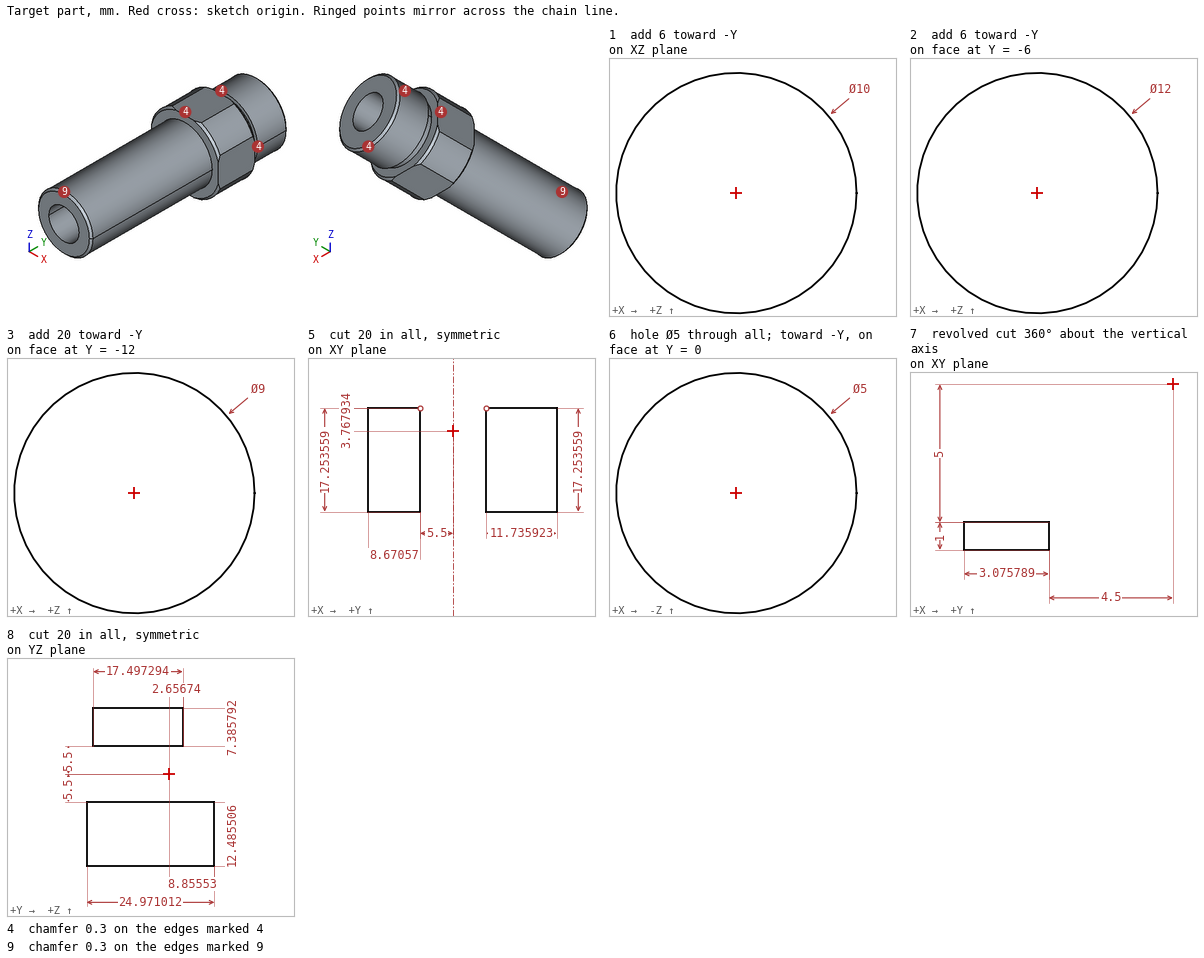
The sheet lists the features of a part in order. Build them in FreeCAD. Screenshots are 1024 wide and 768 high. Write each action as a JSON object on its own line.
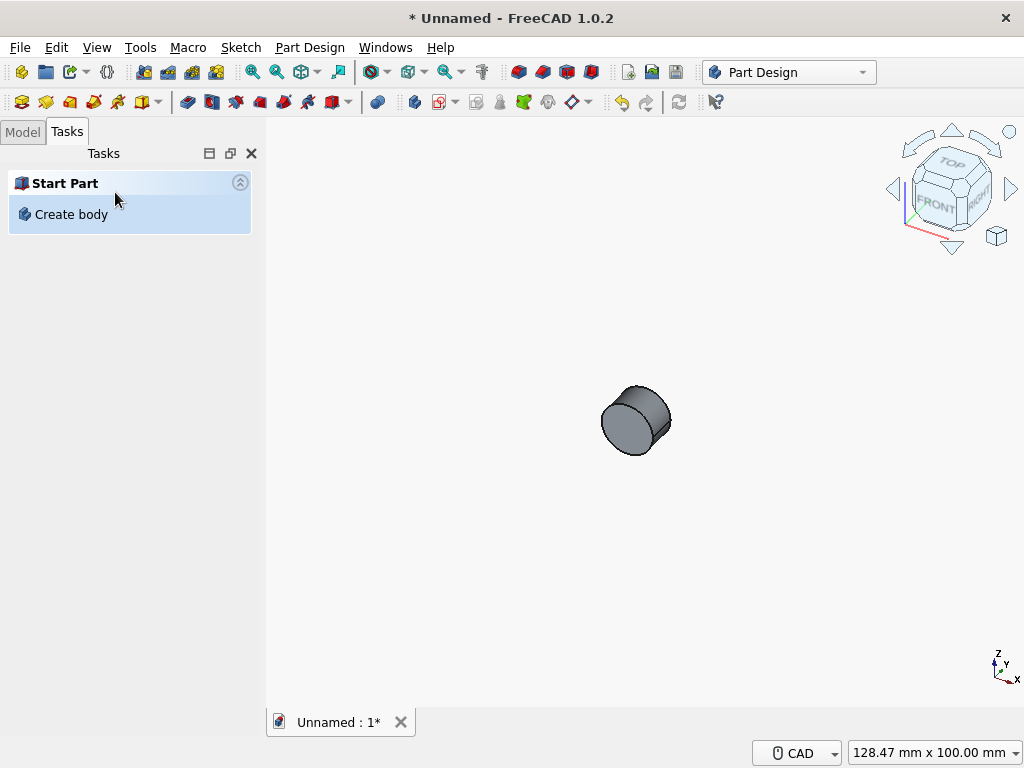
{"action": "key", "text": "v f"}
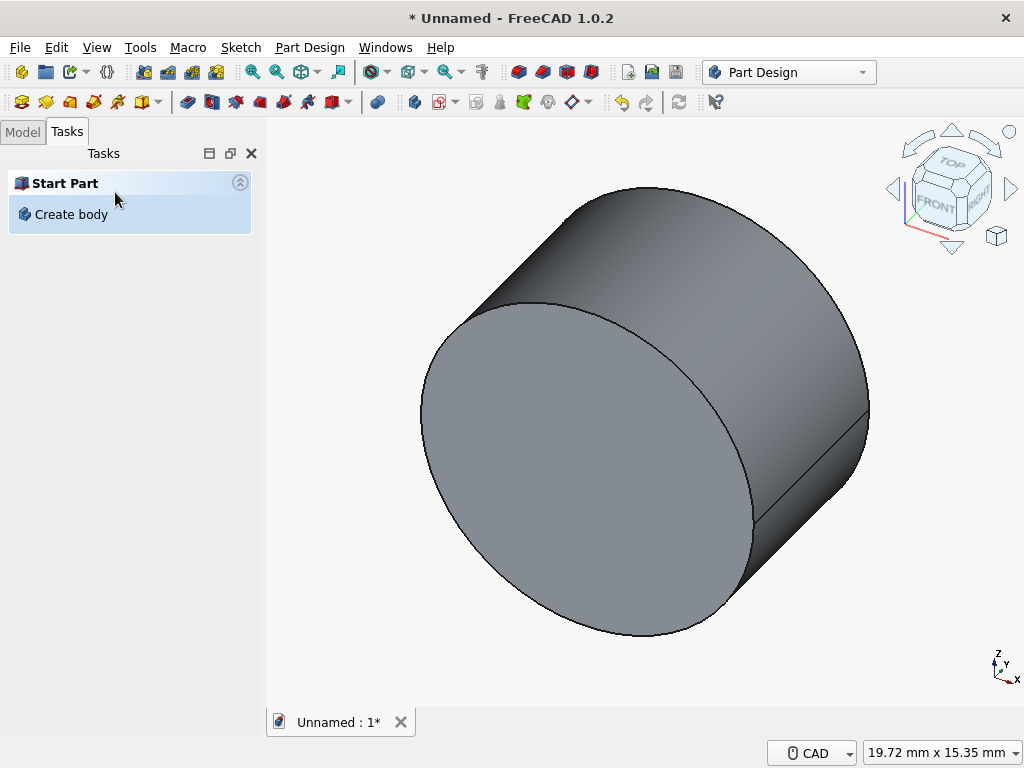
{"action": "left_click", "coordinate": [587, 468]}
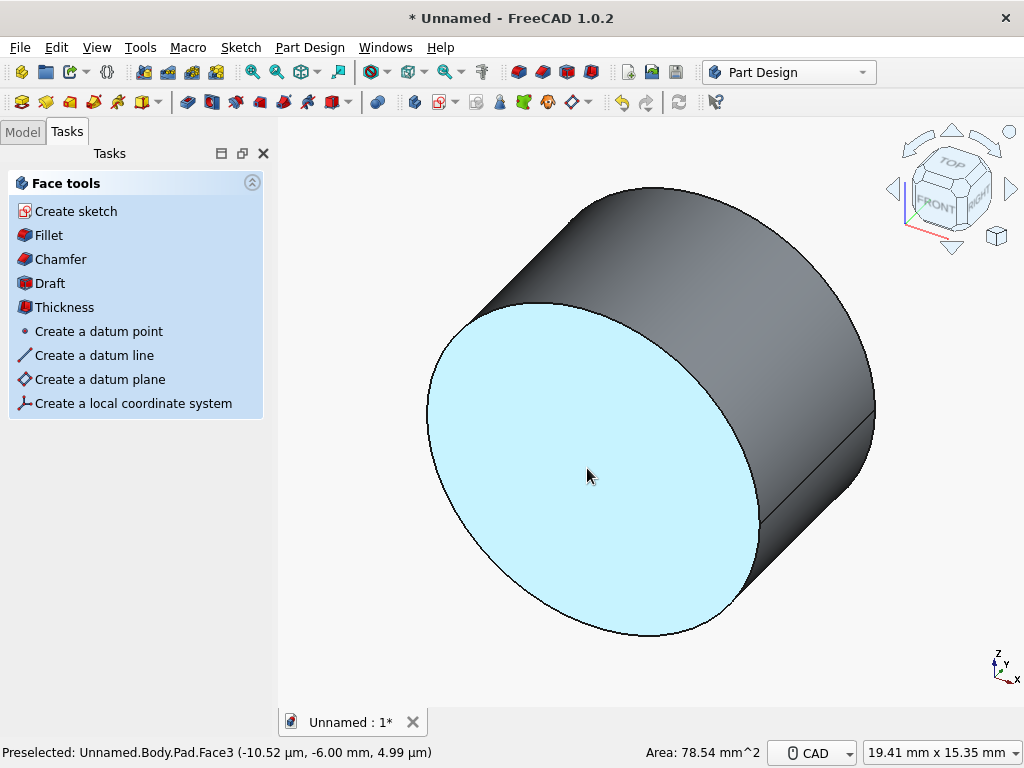
{"action": "left_click", "coordinate": [440, 102]}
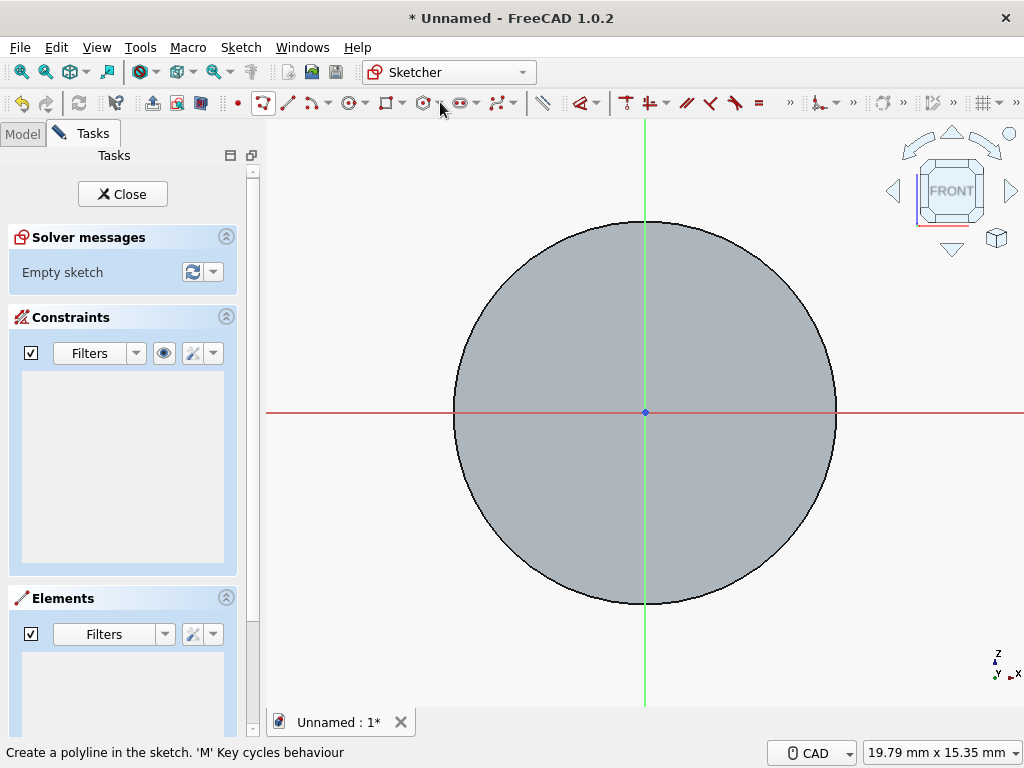
{"action": "scroll", "coordinate": [294, 413], "scroll_direction": "down", "scroll_amount": 1}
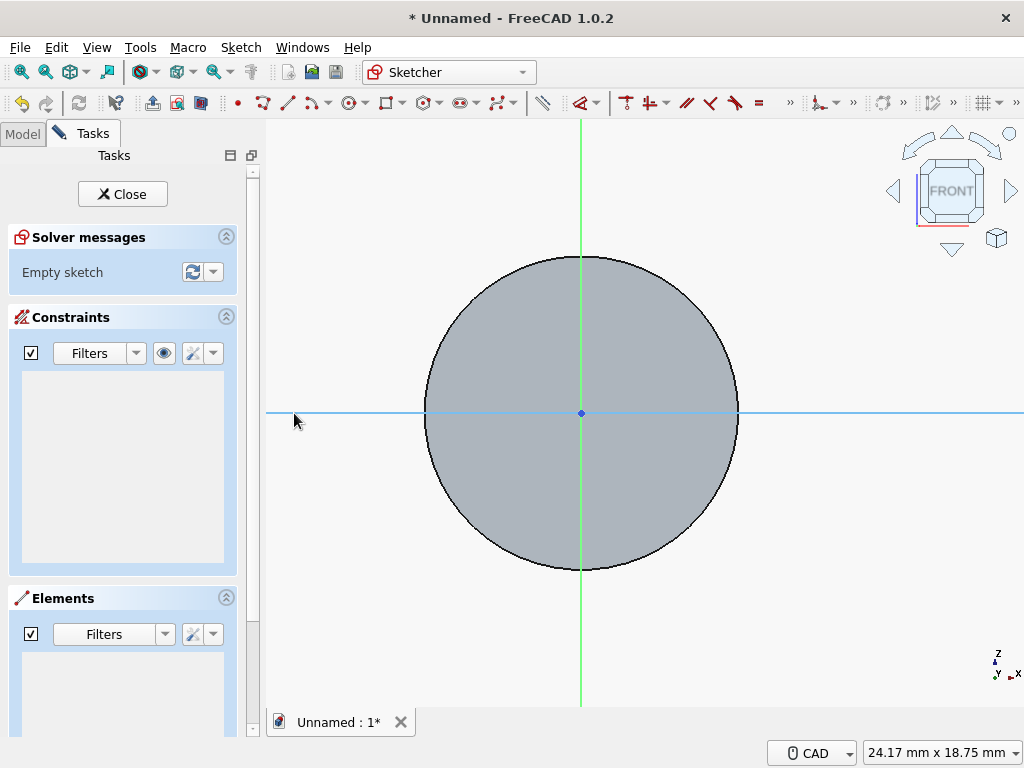
{"action": "left_click", "coordinate": [350, 104]}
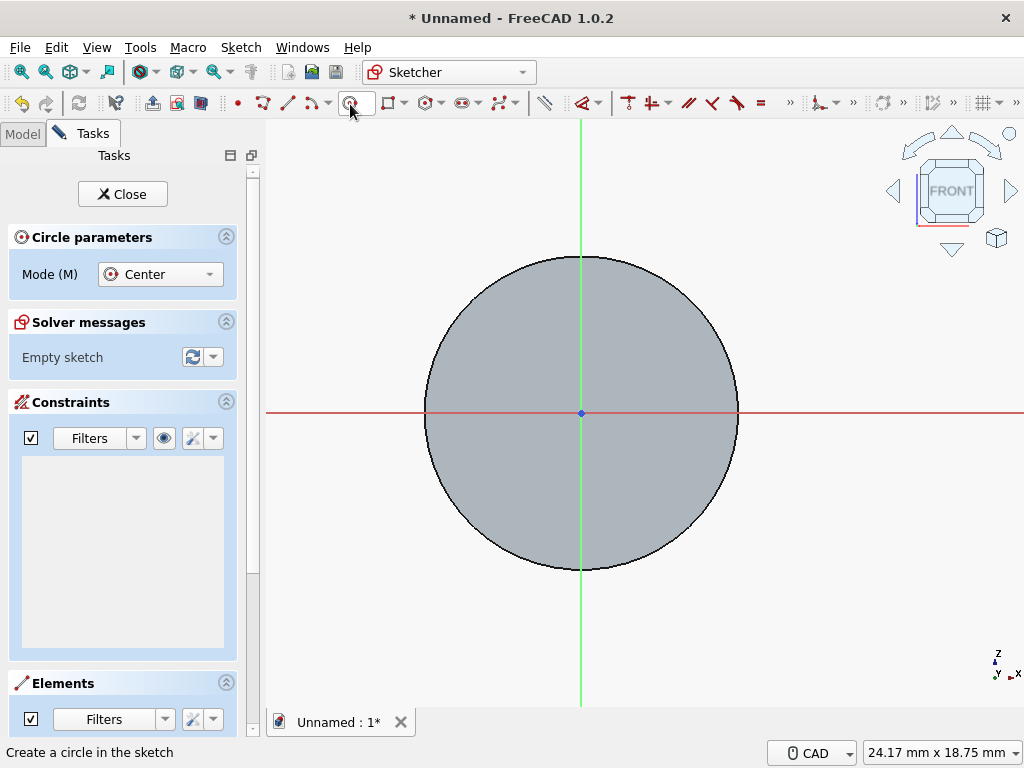
{"action": "left_click", "coordinate": [581, 413]}
{"action": "mouse_move", "coordinate": [714, 280]}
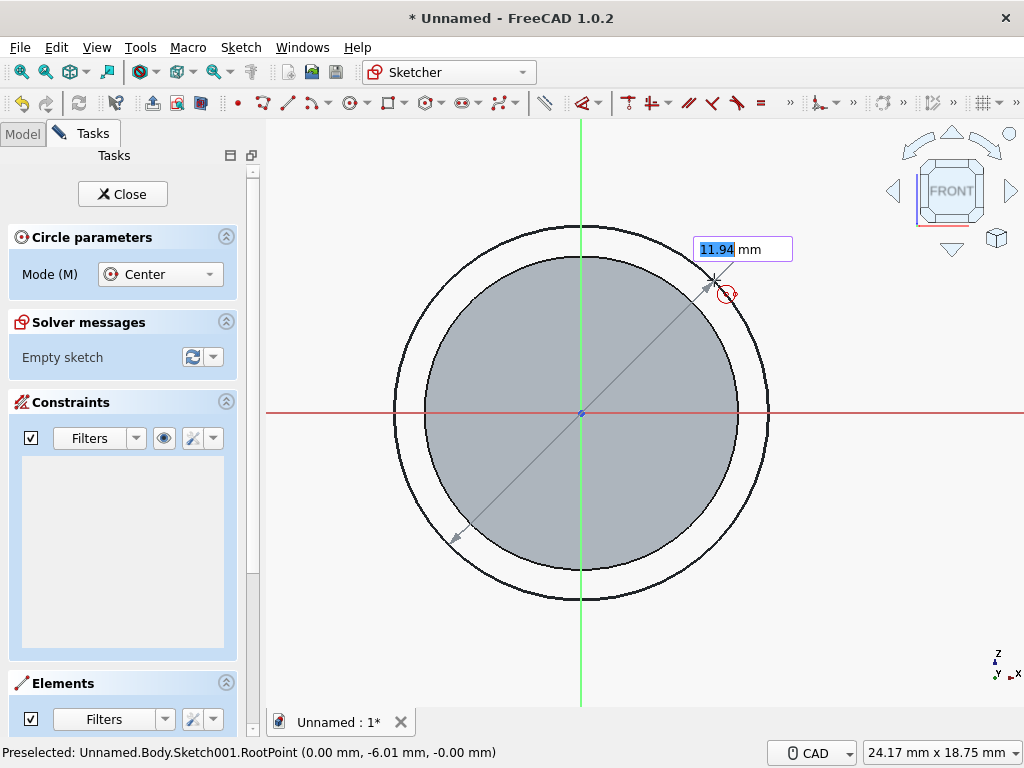
{"action": "type", "text": "12"}
{"action": "key", "text": "Return"}
{"action": "key", "text": "Escape"}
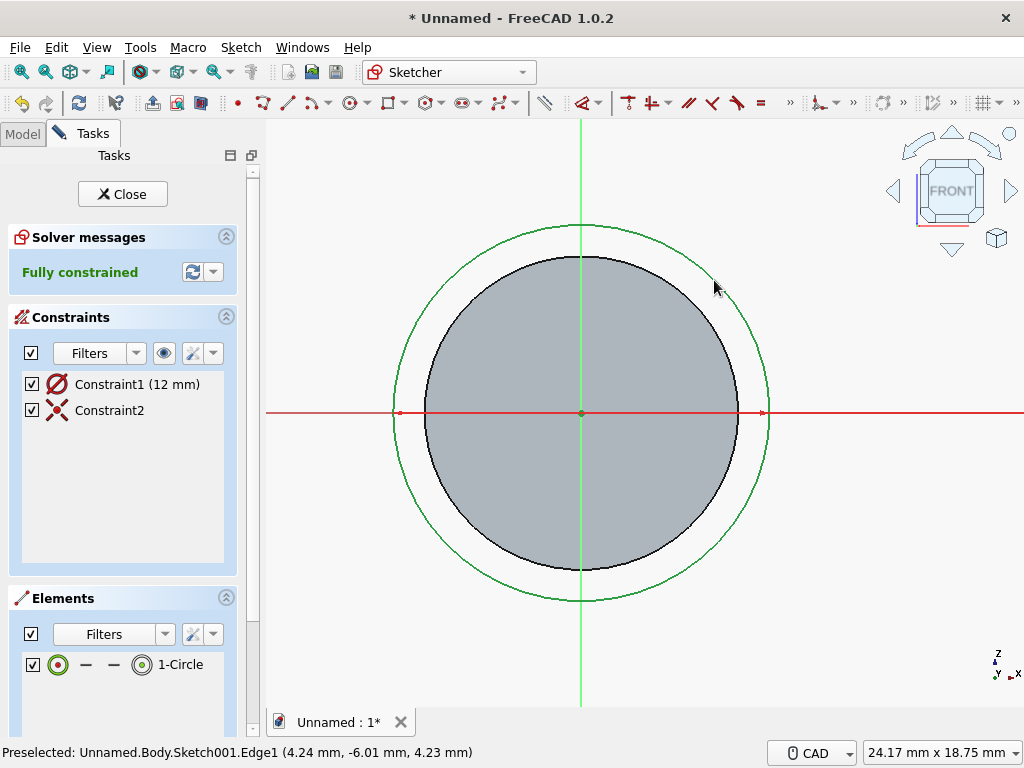
{"action": "left_click", "coordinate": [123, 194]}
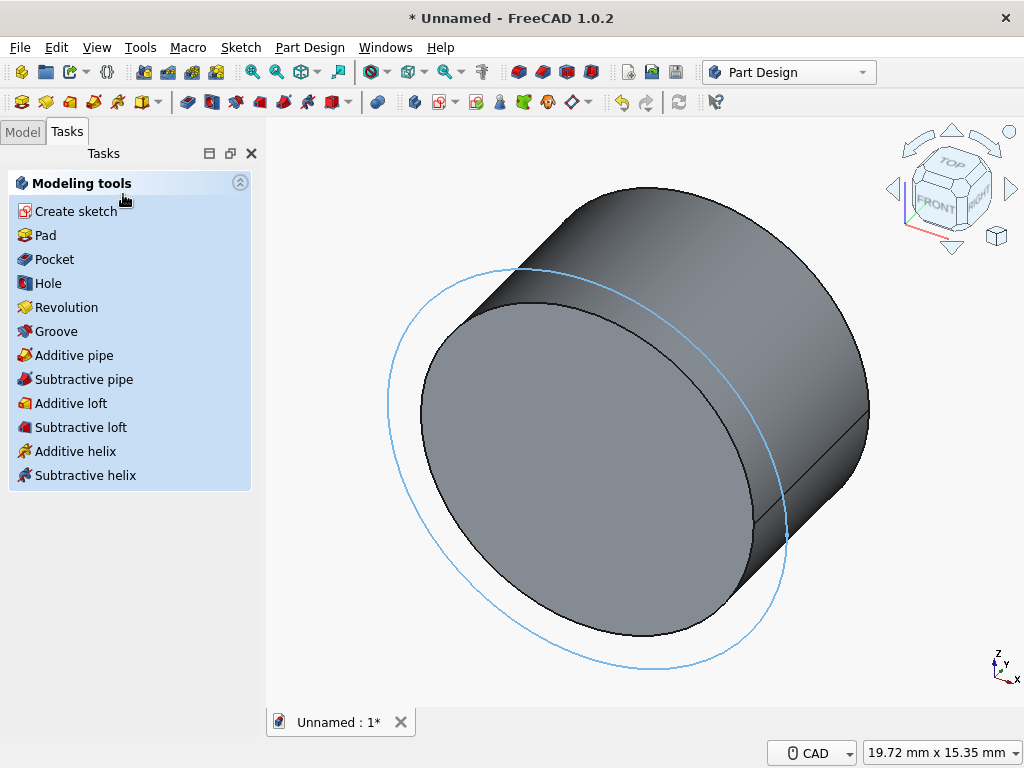
{"action": "left_click", "coordinate": [22, 102]}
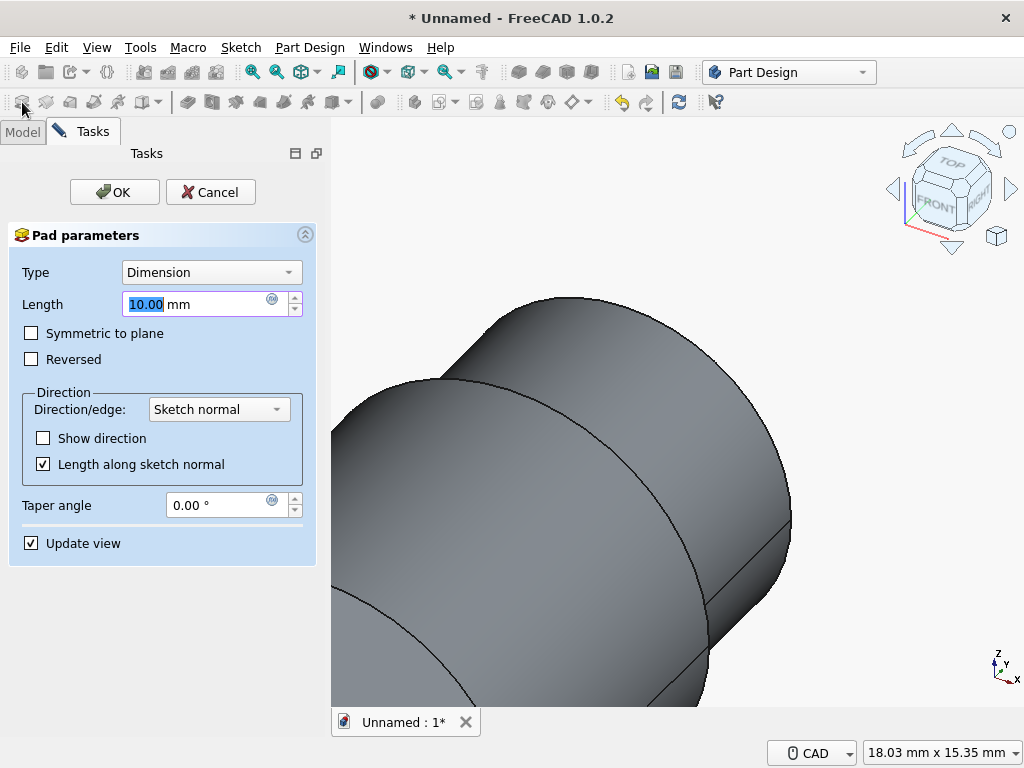
{"action": "type", "text": "6"}
{"action": "key", "text": "Tab"}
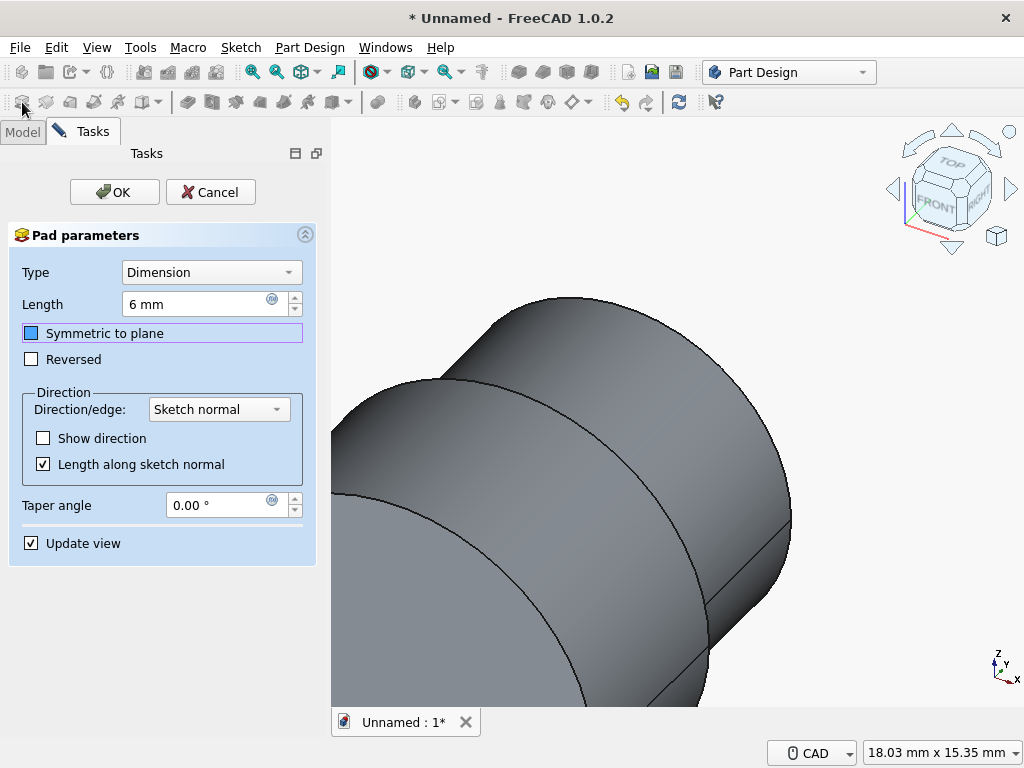
{"action": "left_click", "coordinate": [115, 192]}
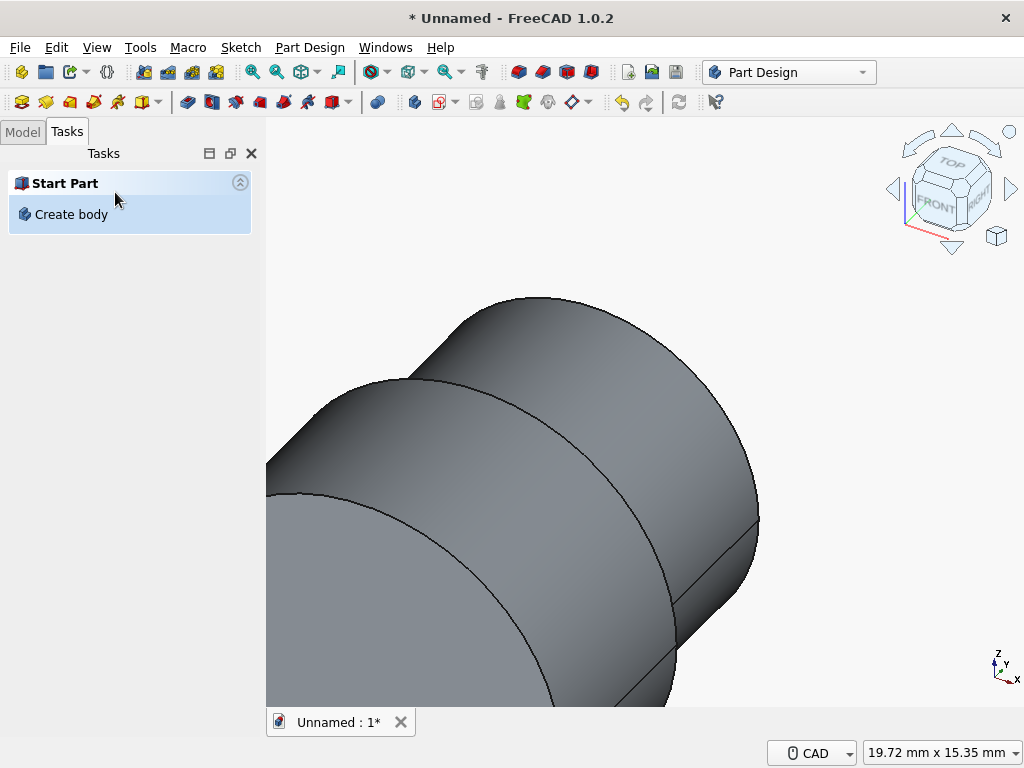
{"action": "left_click", "coordinate": [254, 72]}